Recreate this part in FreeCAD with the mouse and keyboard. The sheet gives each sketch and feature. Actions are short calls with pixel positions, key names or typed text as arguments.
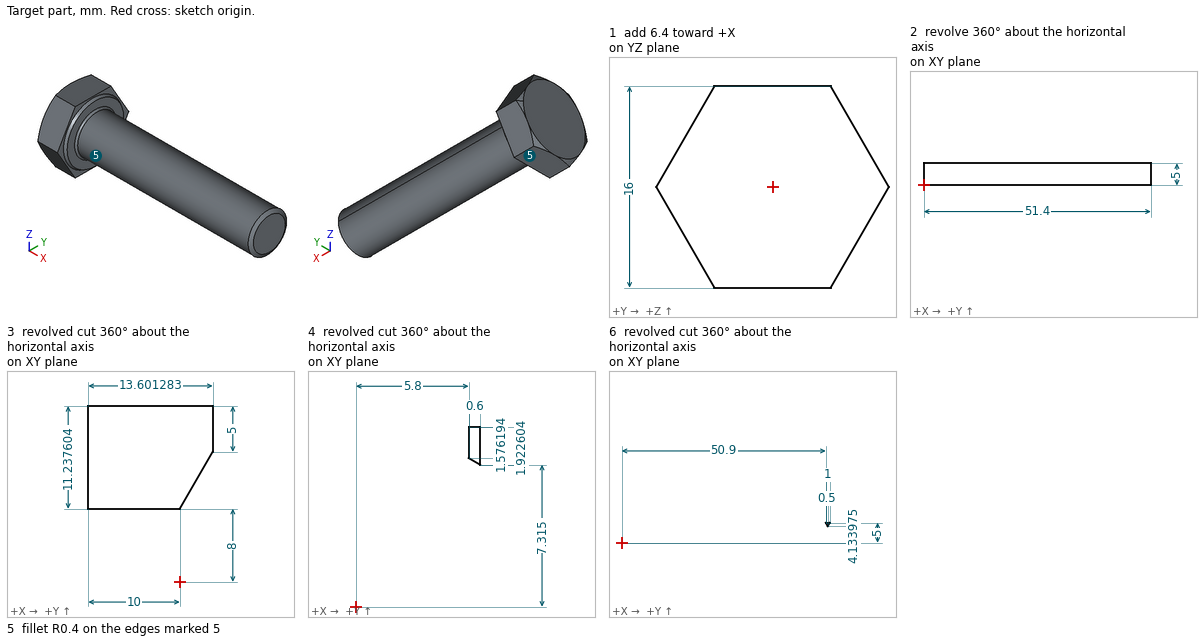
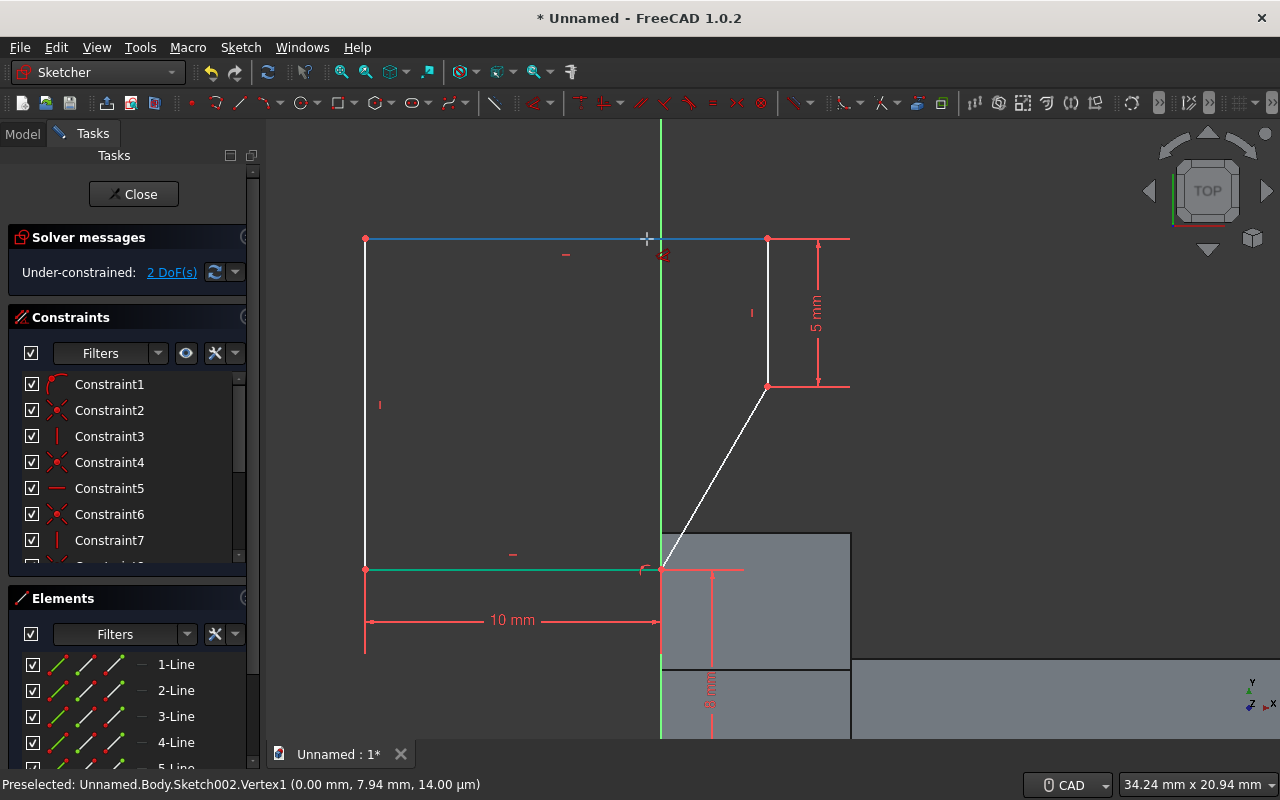
click(647, 239)
click(566, 205)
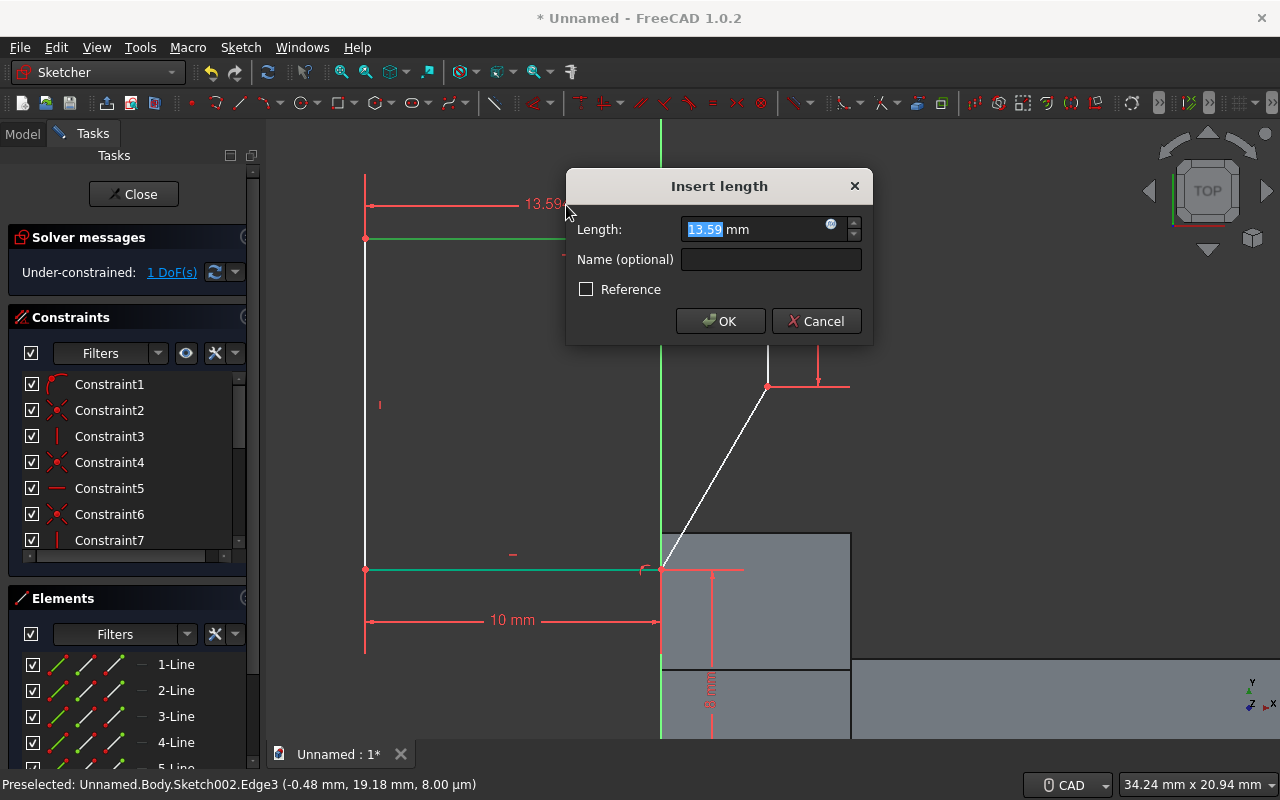
text(13.601283)
key(Return)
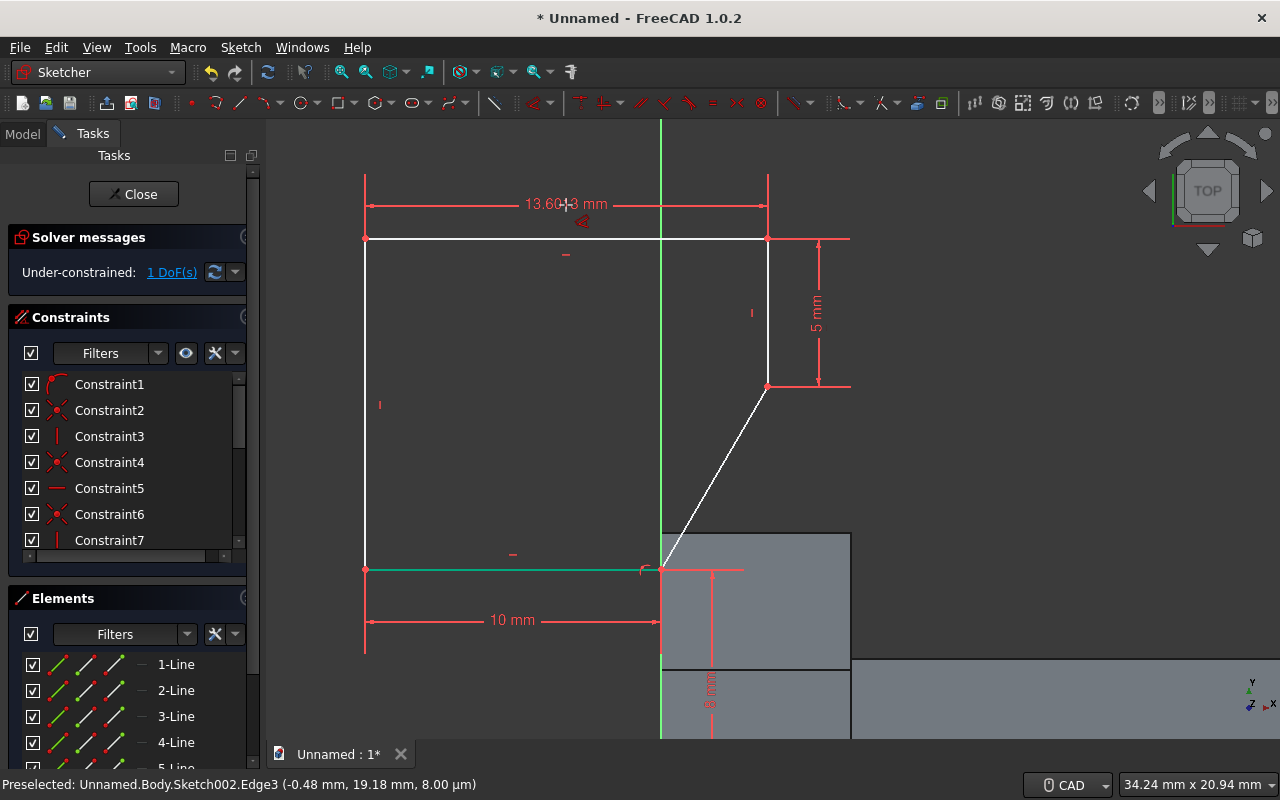
click(365, 338)
click(331, 404)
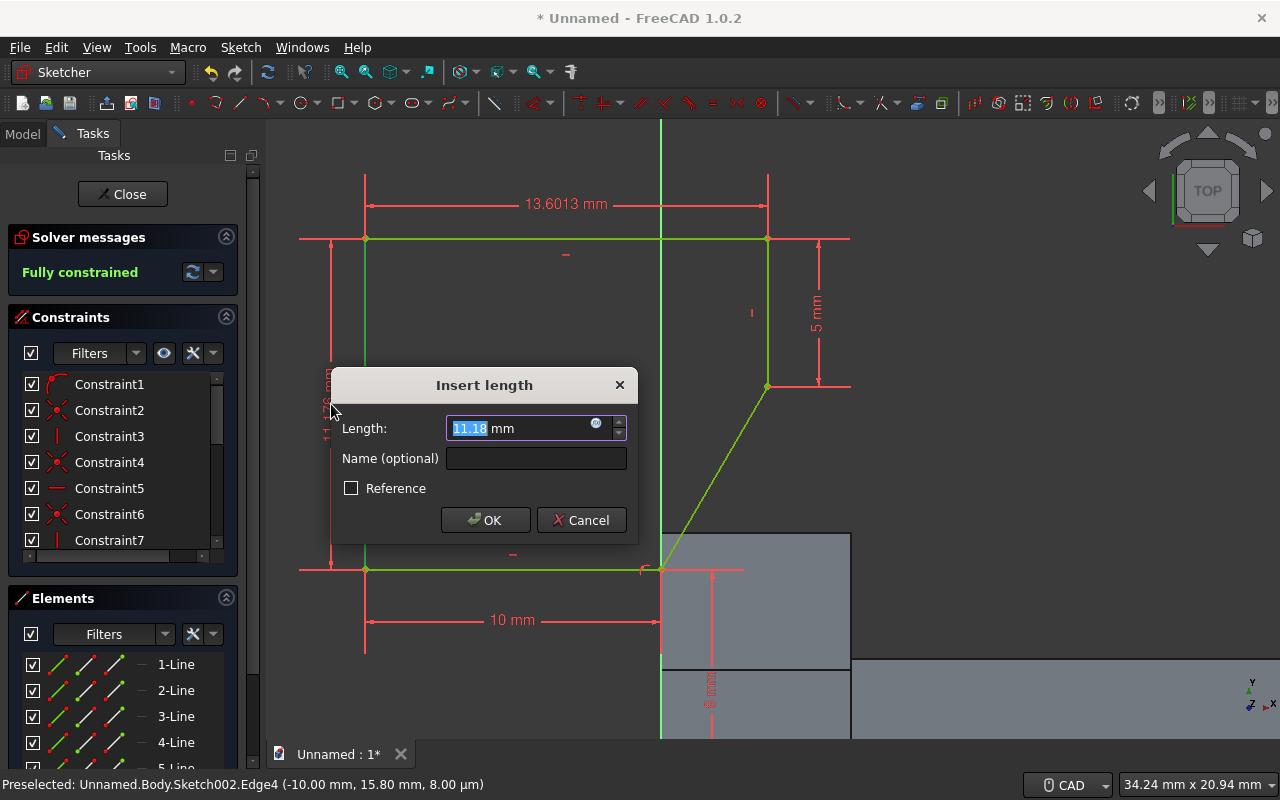
text(11.237604)
key(Return)
key(Escape)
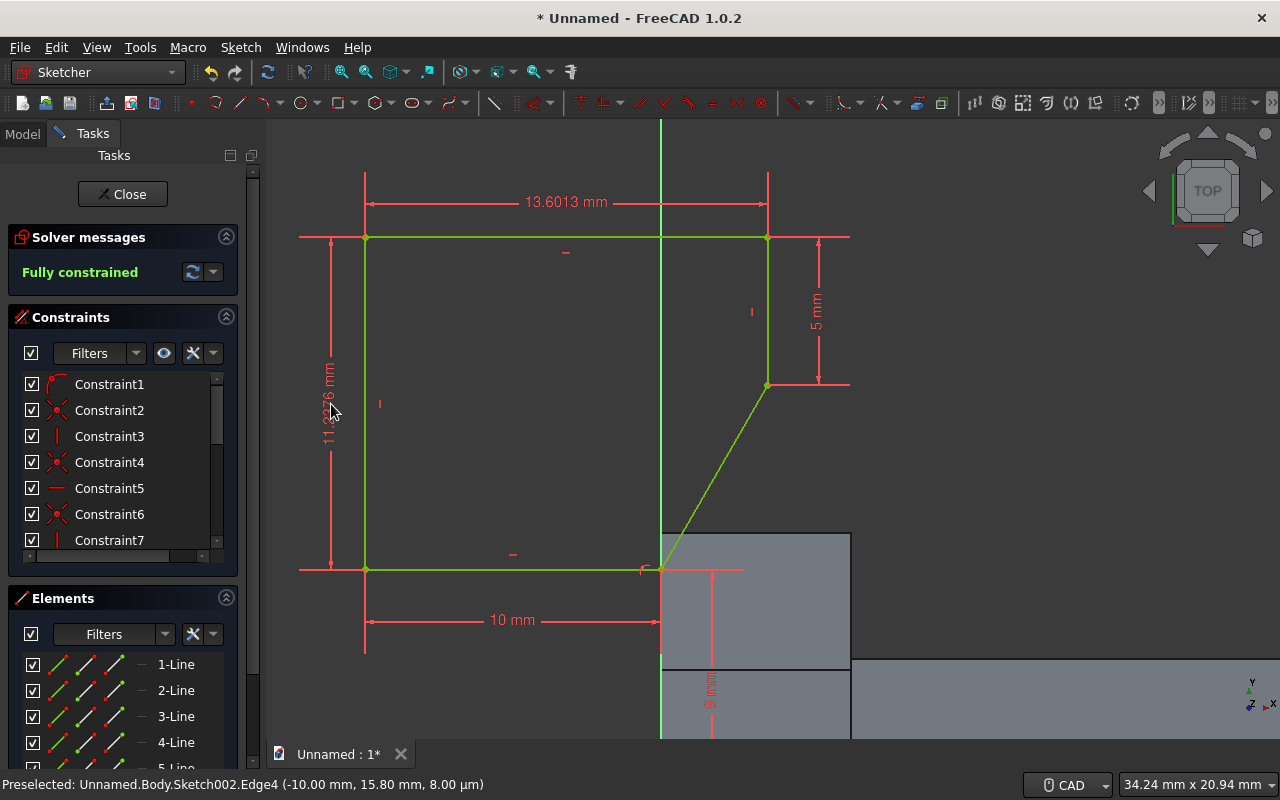
click(123, 194)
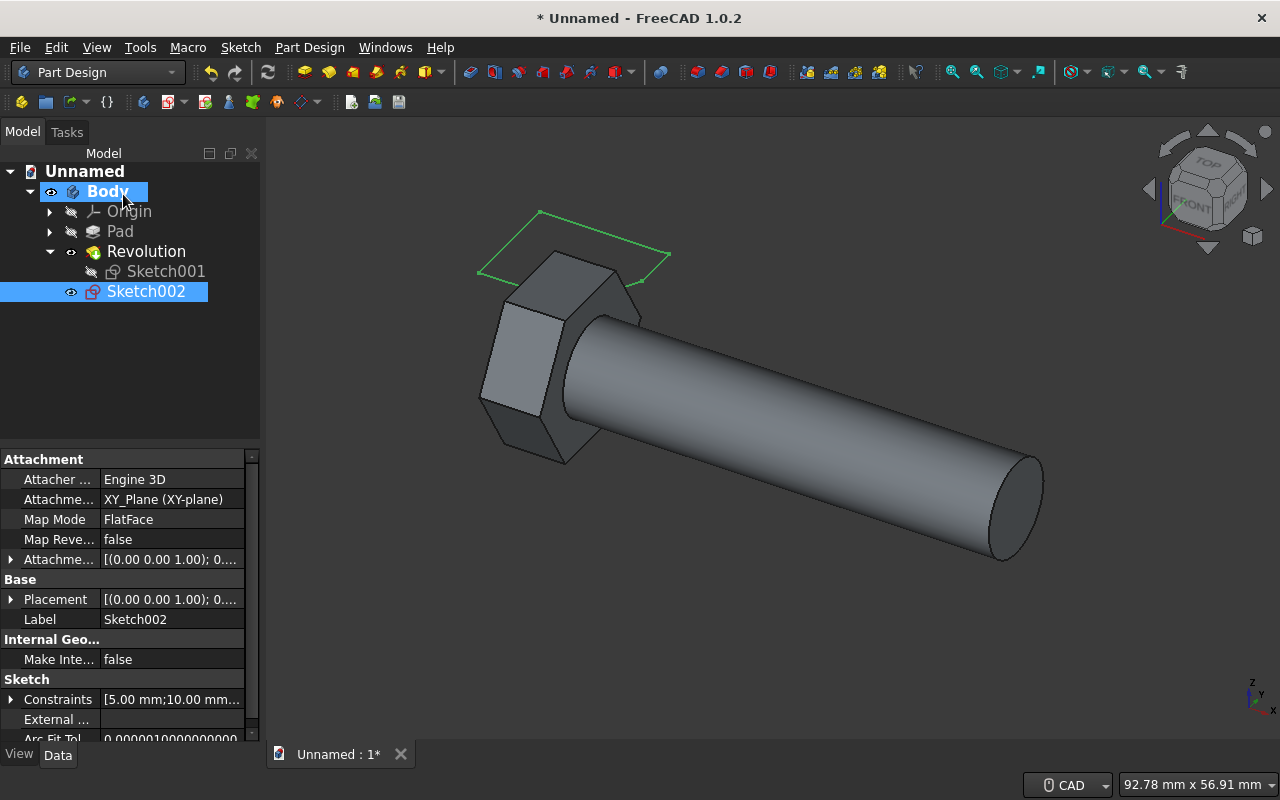
click(520, 72)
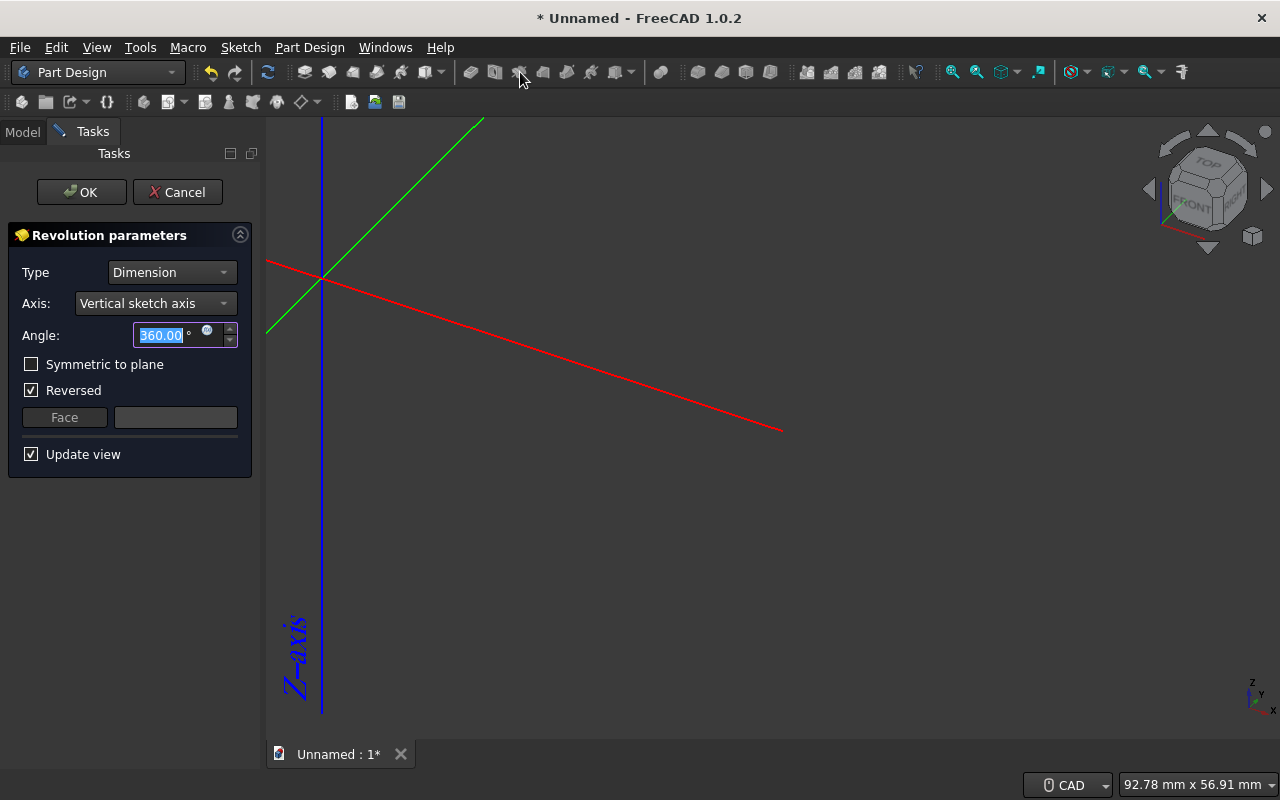
click(156, 304)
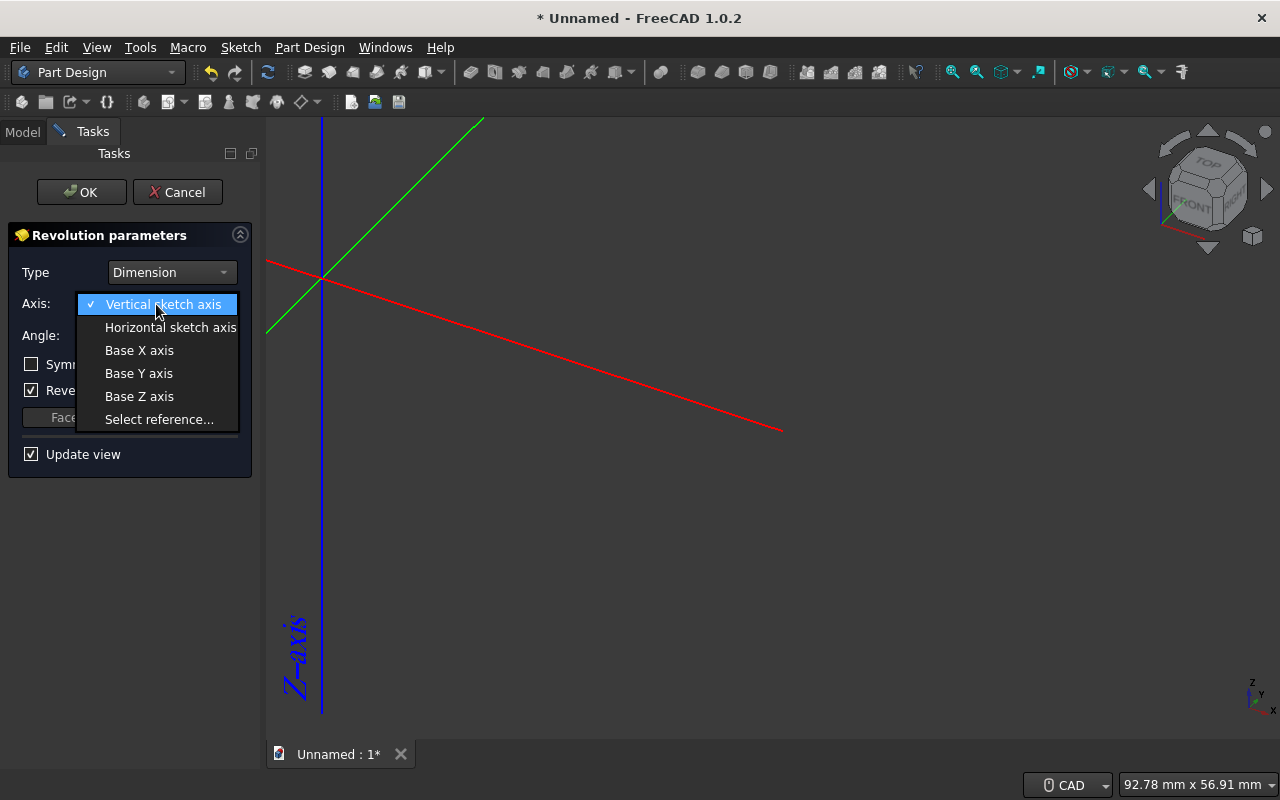
click(156, 328)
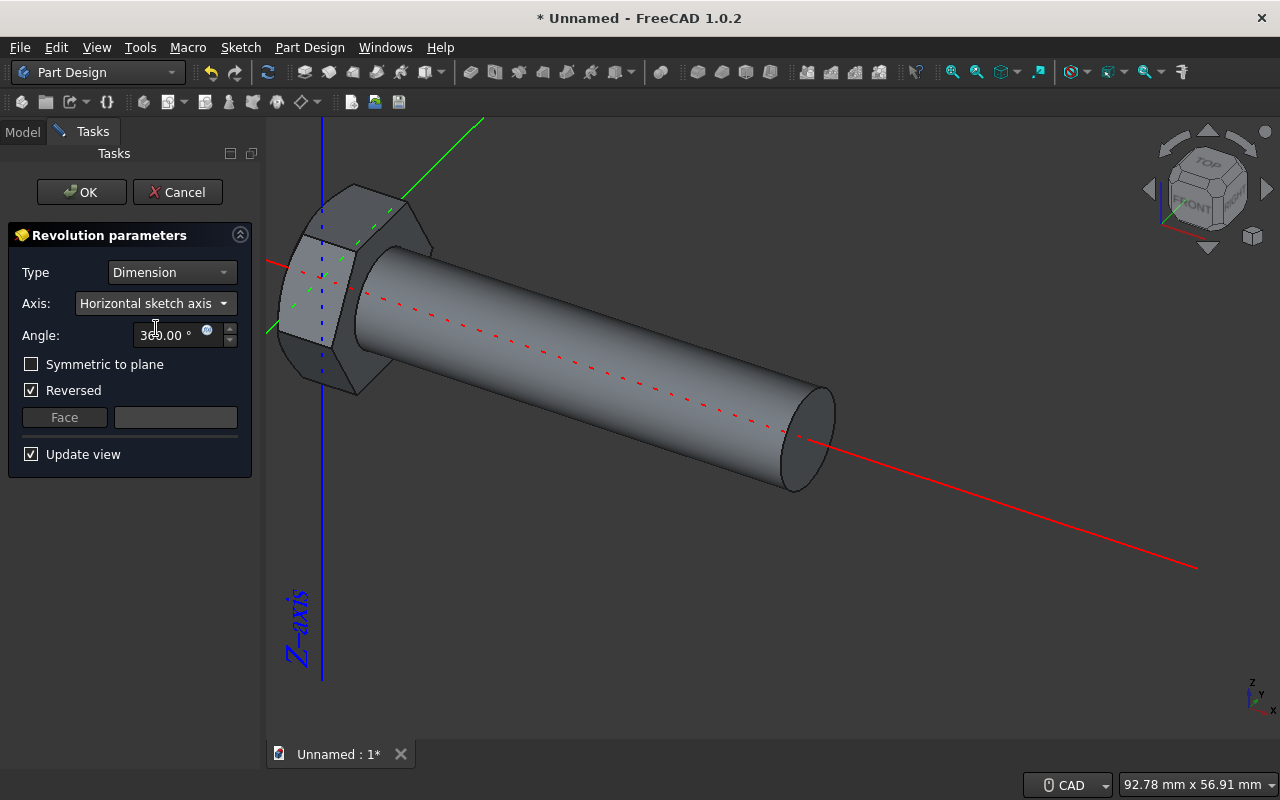
click(82, 192)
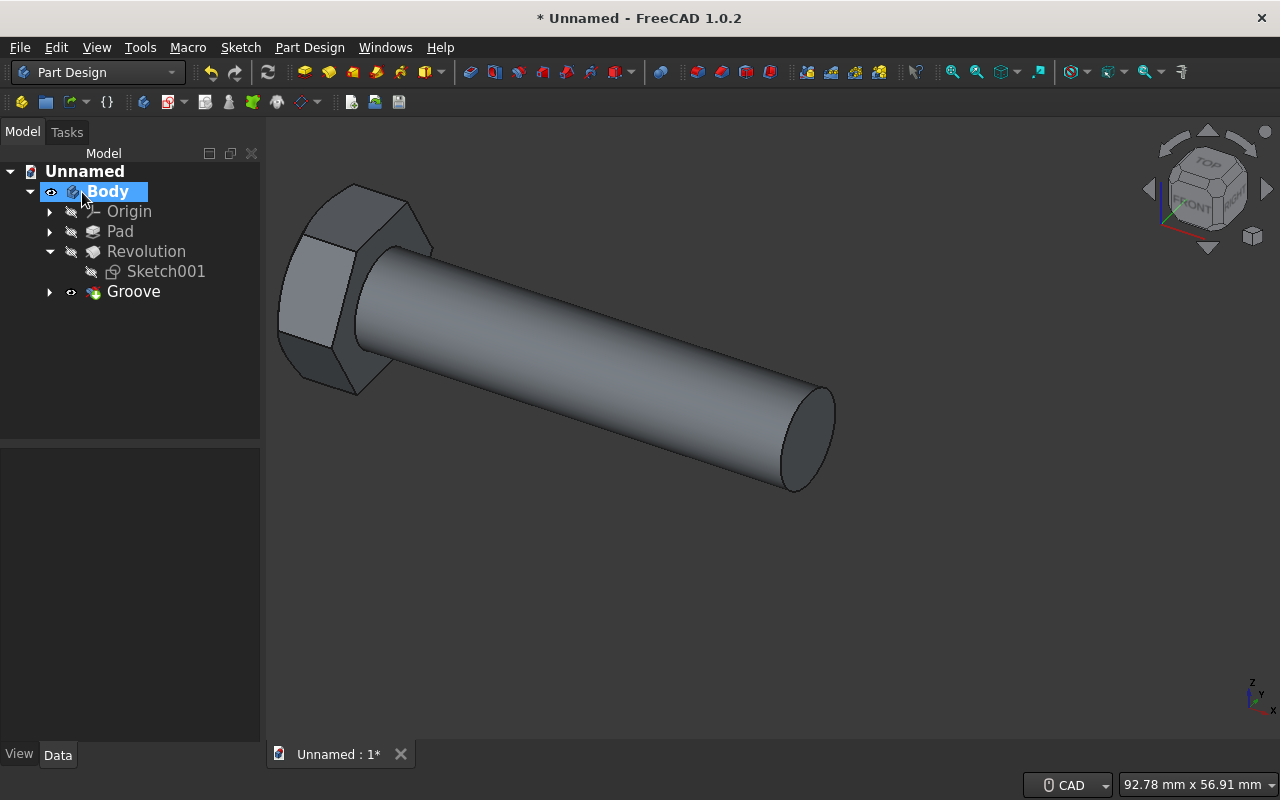
click(168, 102)